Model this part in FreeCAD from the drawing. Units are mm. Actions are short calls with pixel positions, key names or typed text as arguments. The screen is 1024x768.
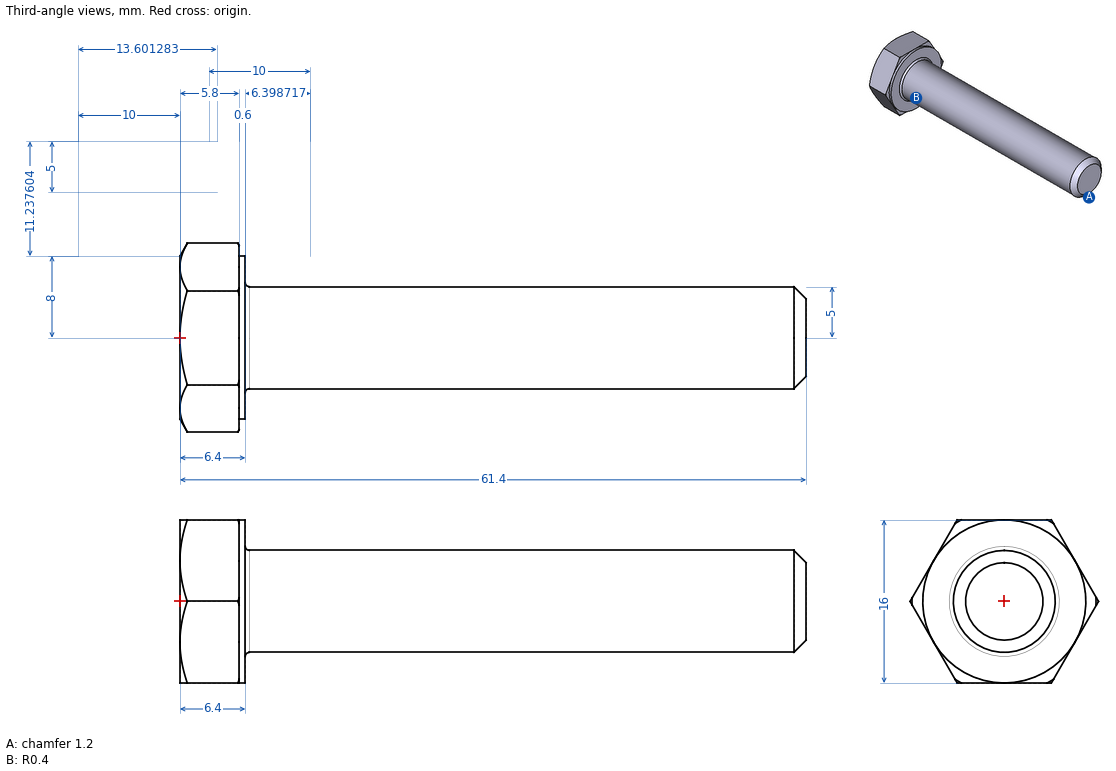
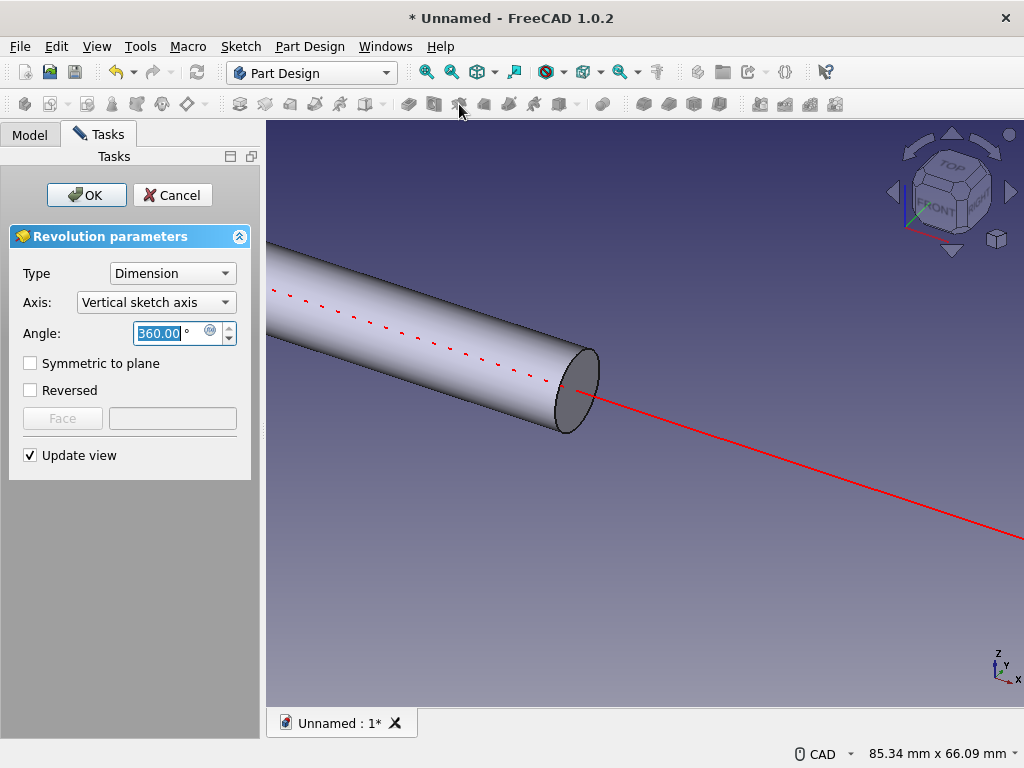
click(157, 302)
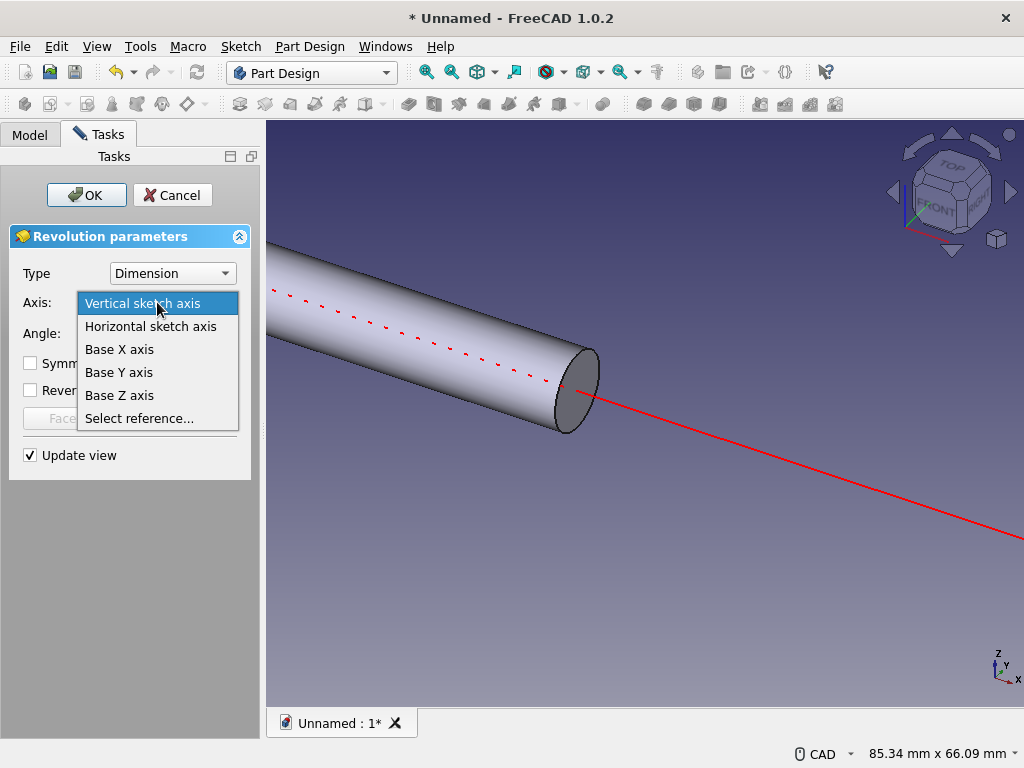
click(156, 326)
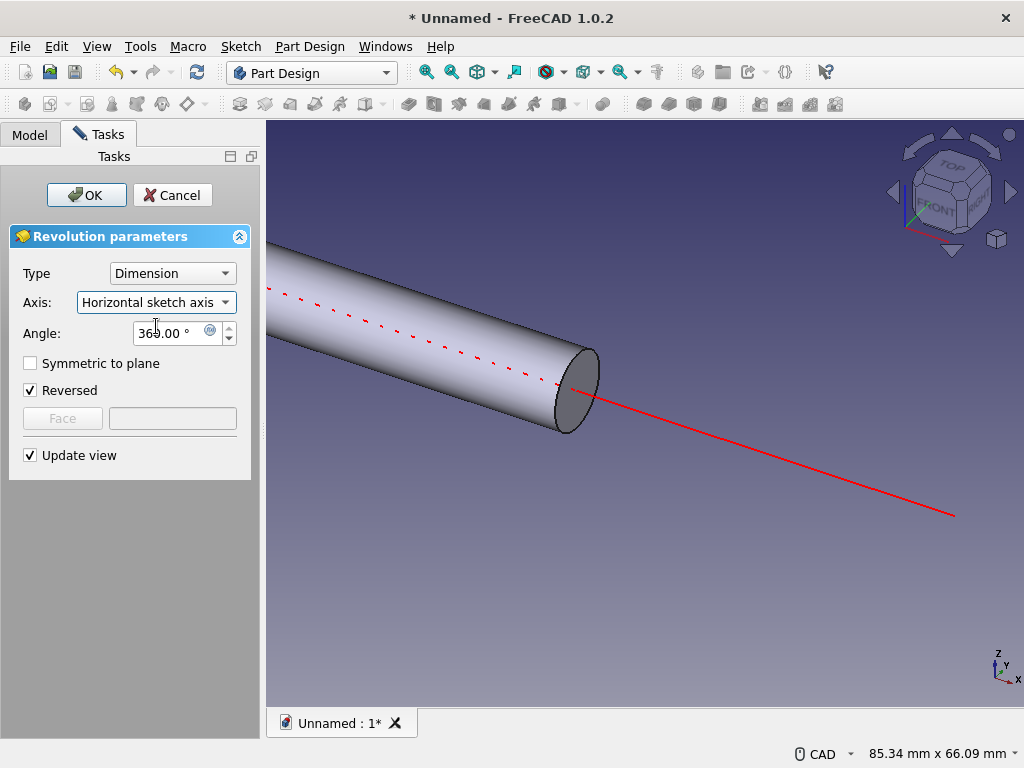
click(87, 195)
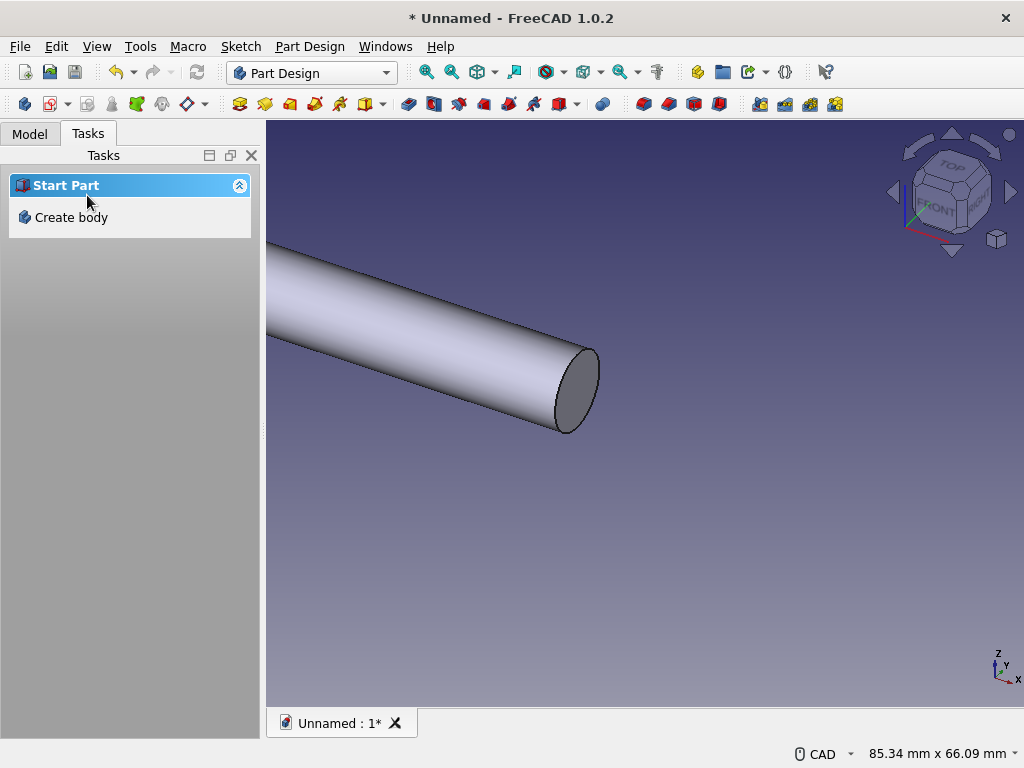
click(427, 72)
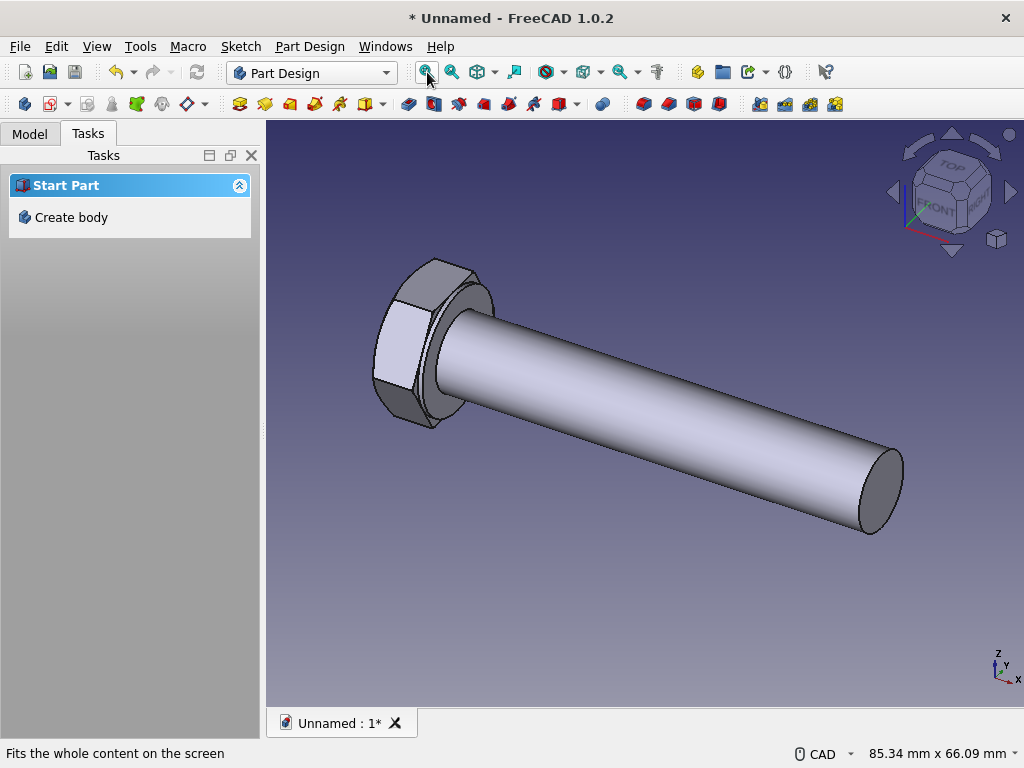
click(859, 513)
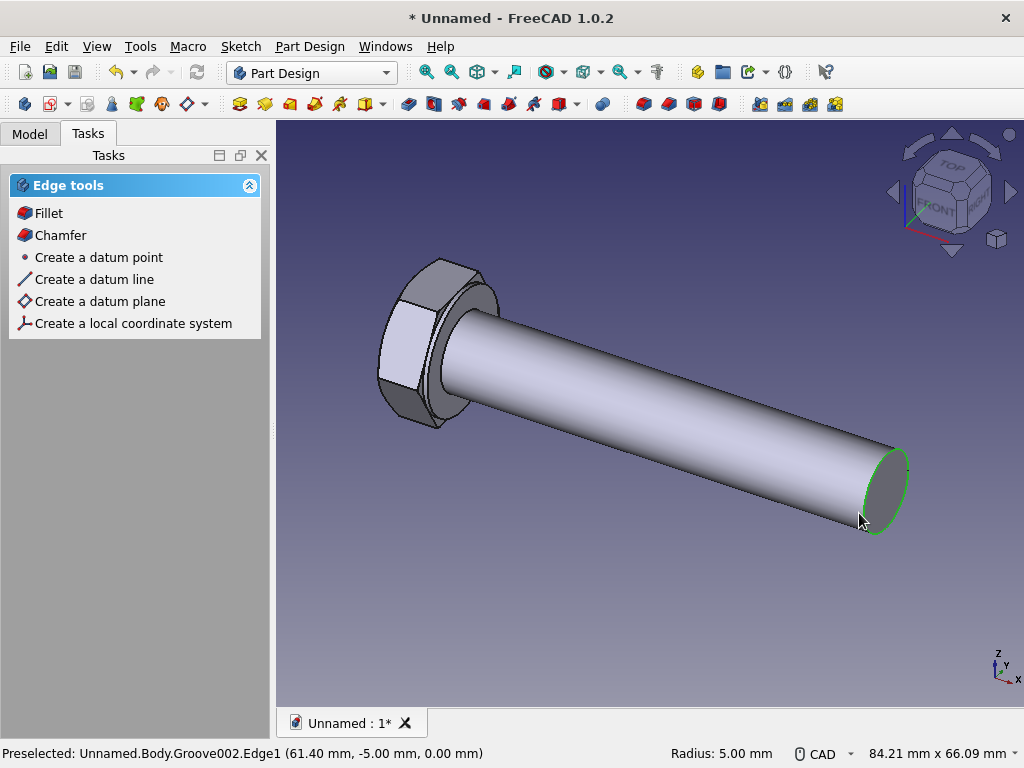
click(669, 104)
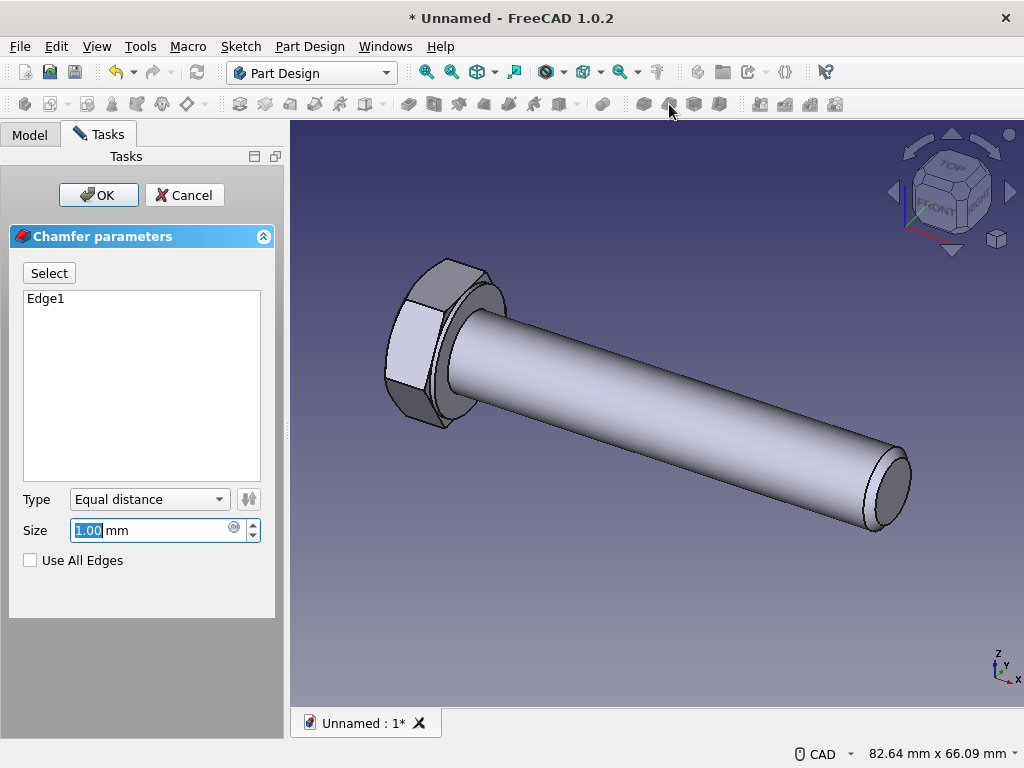
text(1.2)
key(Tab)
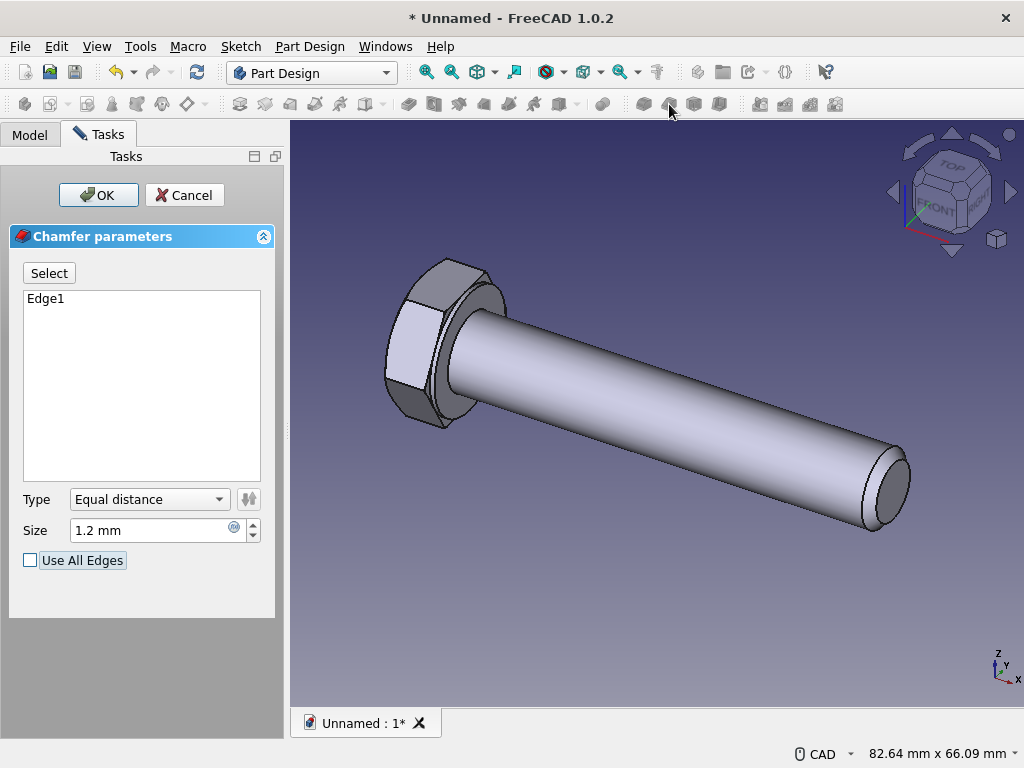
click(99, 195)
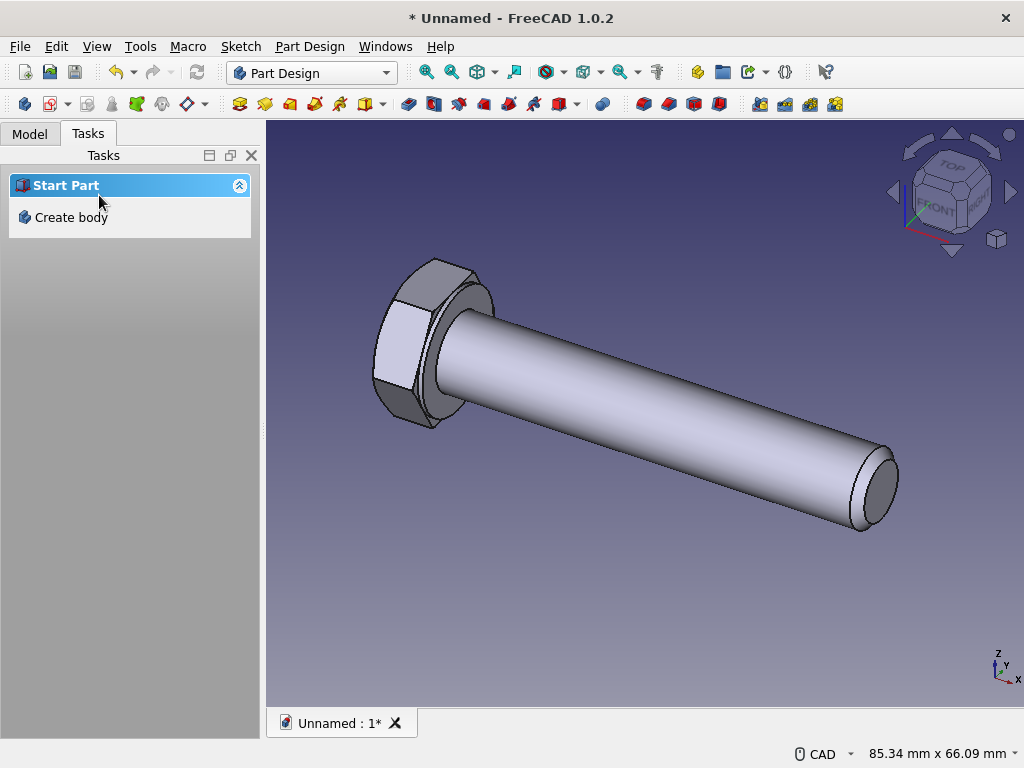
key(0)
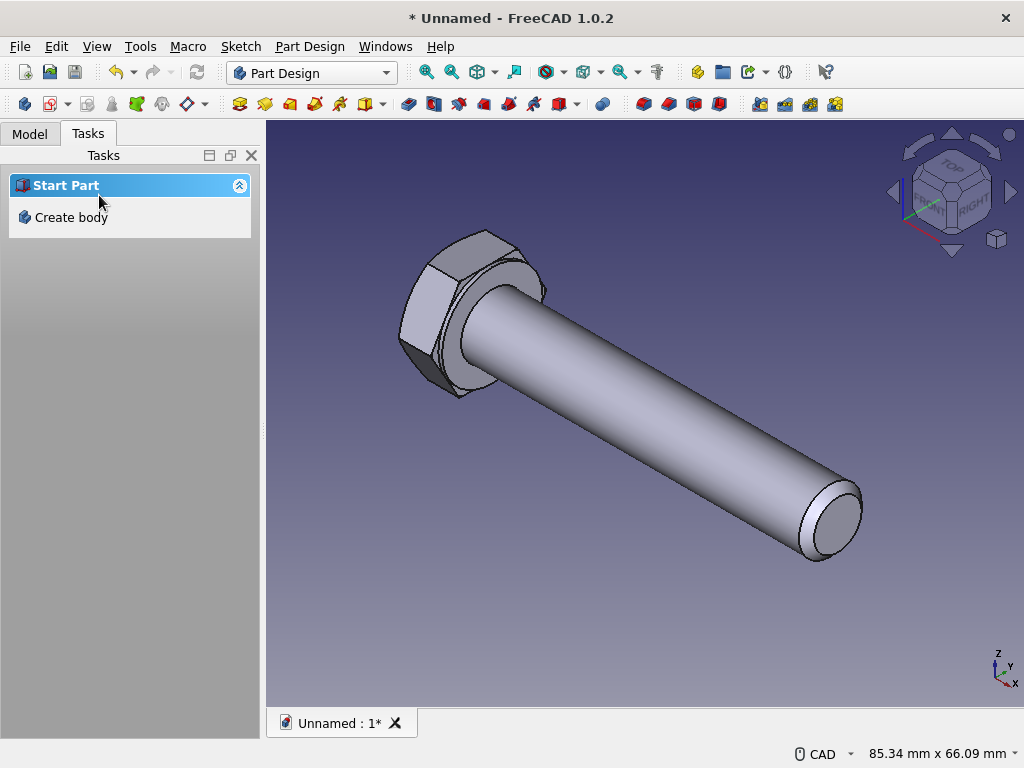
key(2)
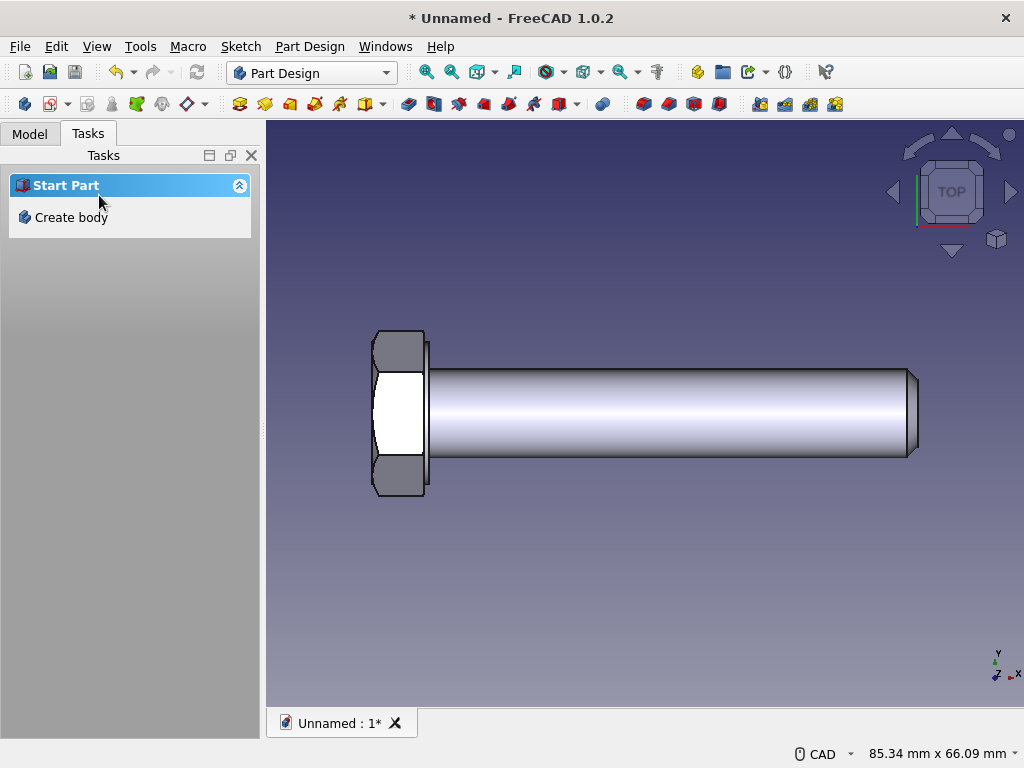
key(1)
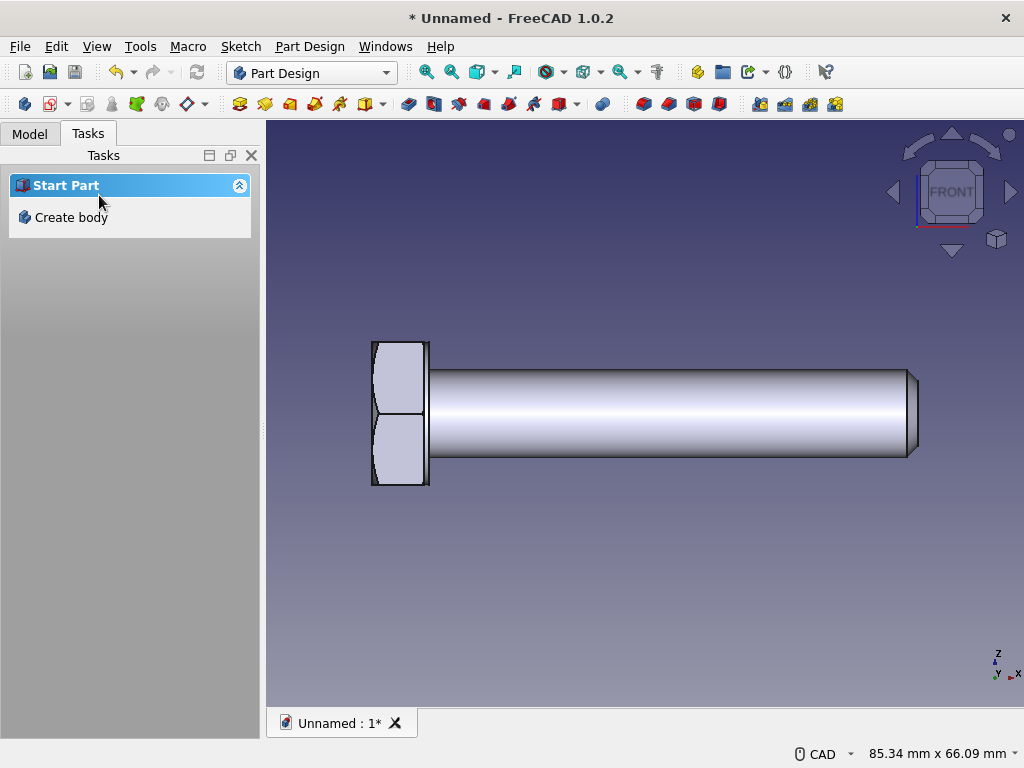
key(3)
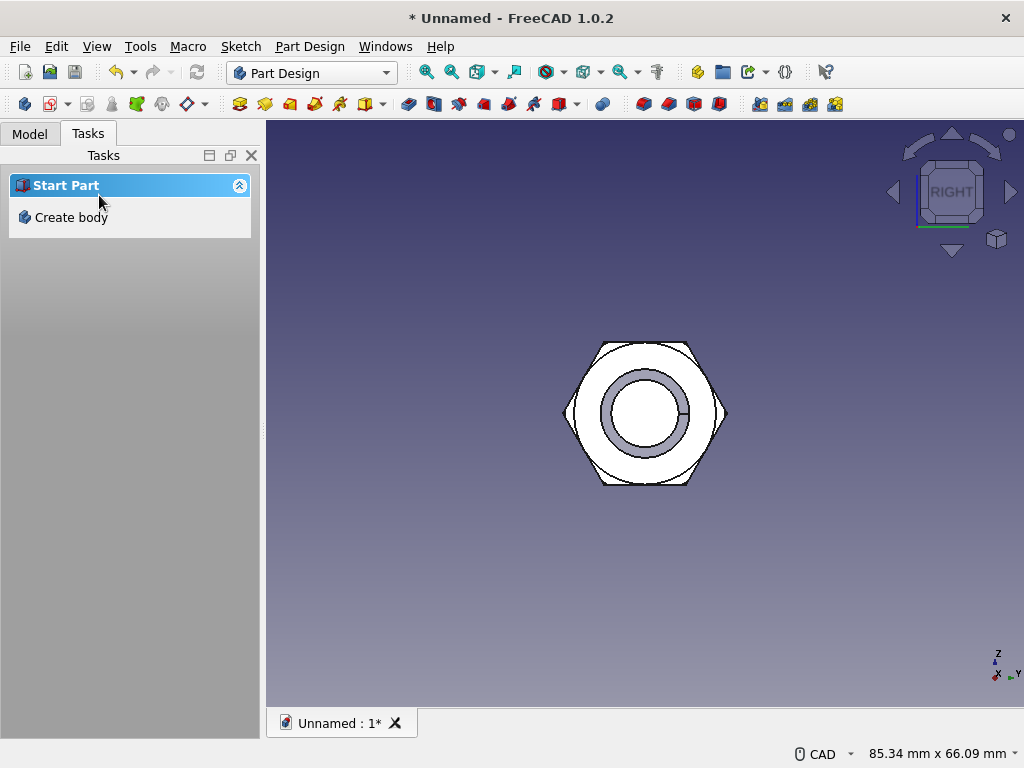
click(427, 72)